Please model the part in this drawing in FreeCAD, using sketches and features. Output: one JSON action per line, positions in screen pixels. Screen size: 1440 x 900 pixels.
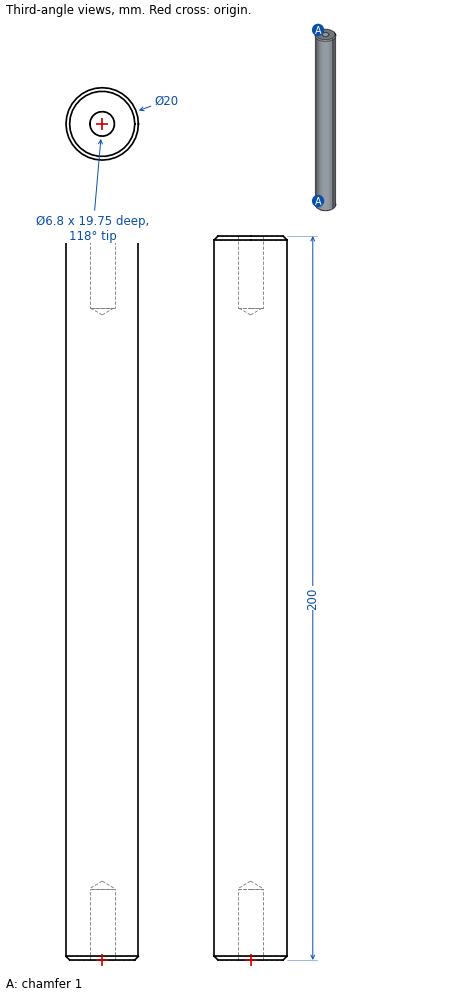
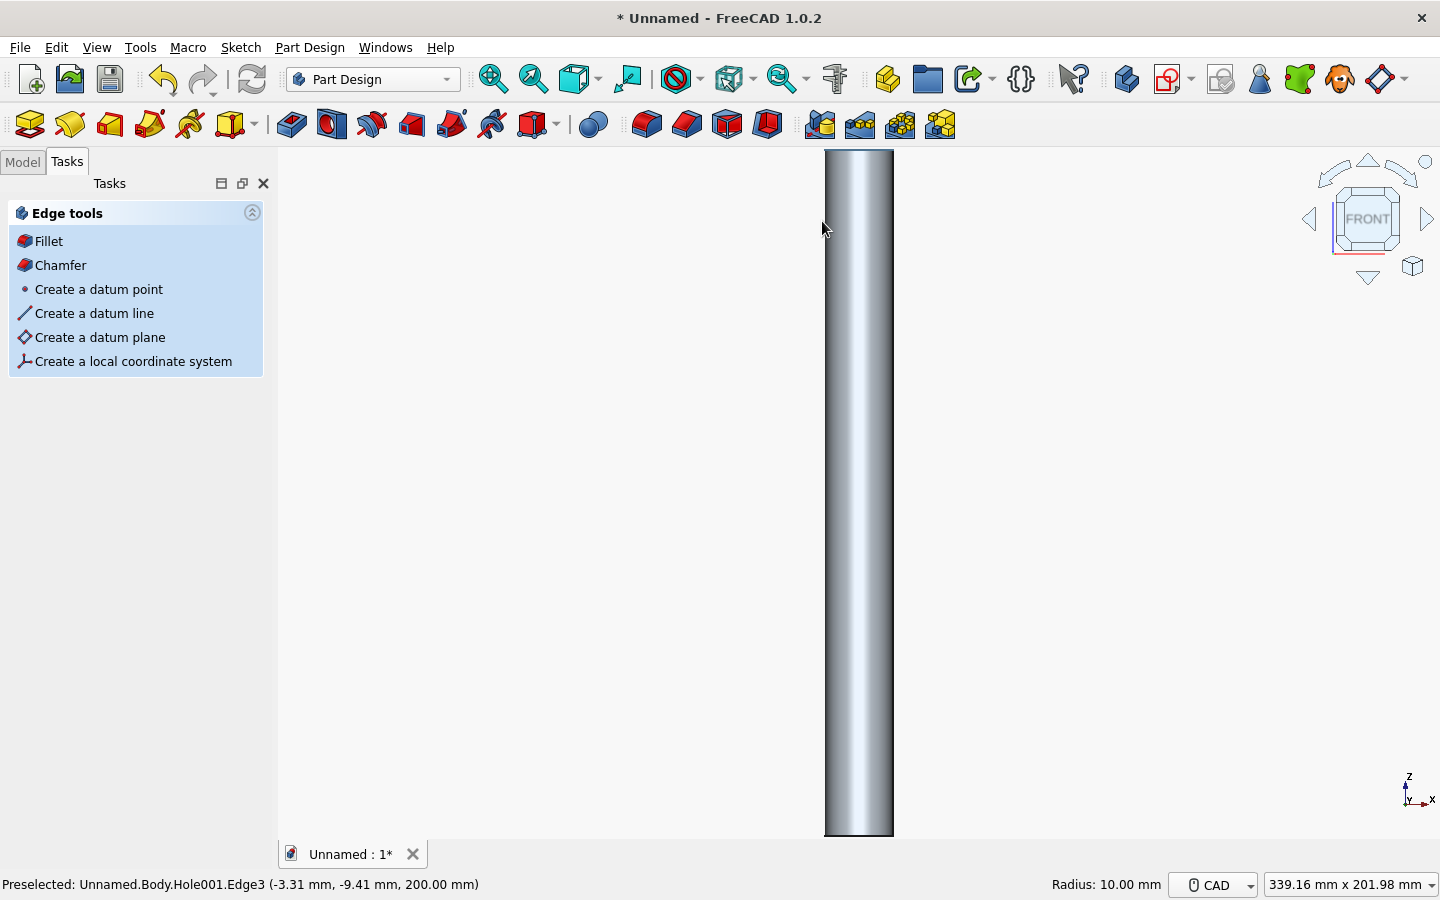
{"action": "key", "text": "3"}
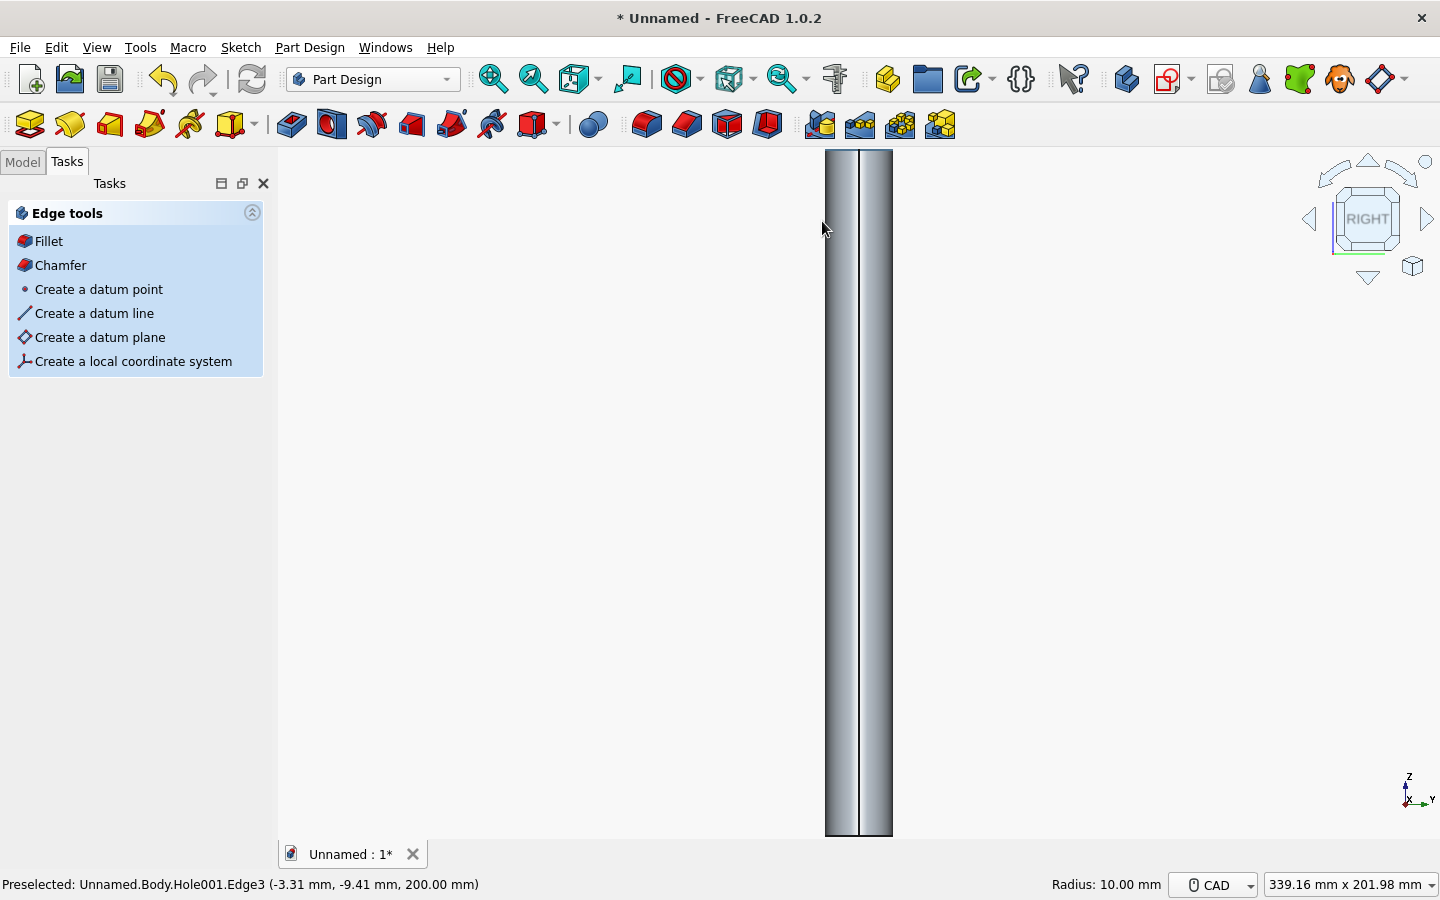
{"action": "key", "text": "5"}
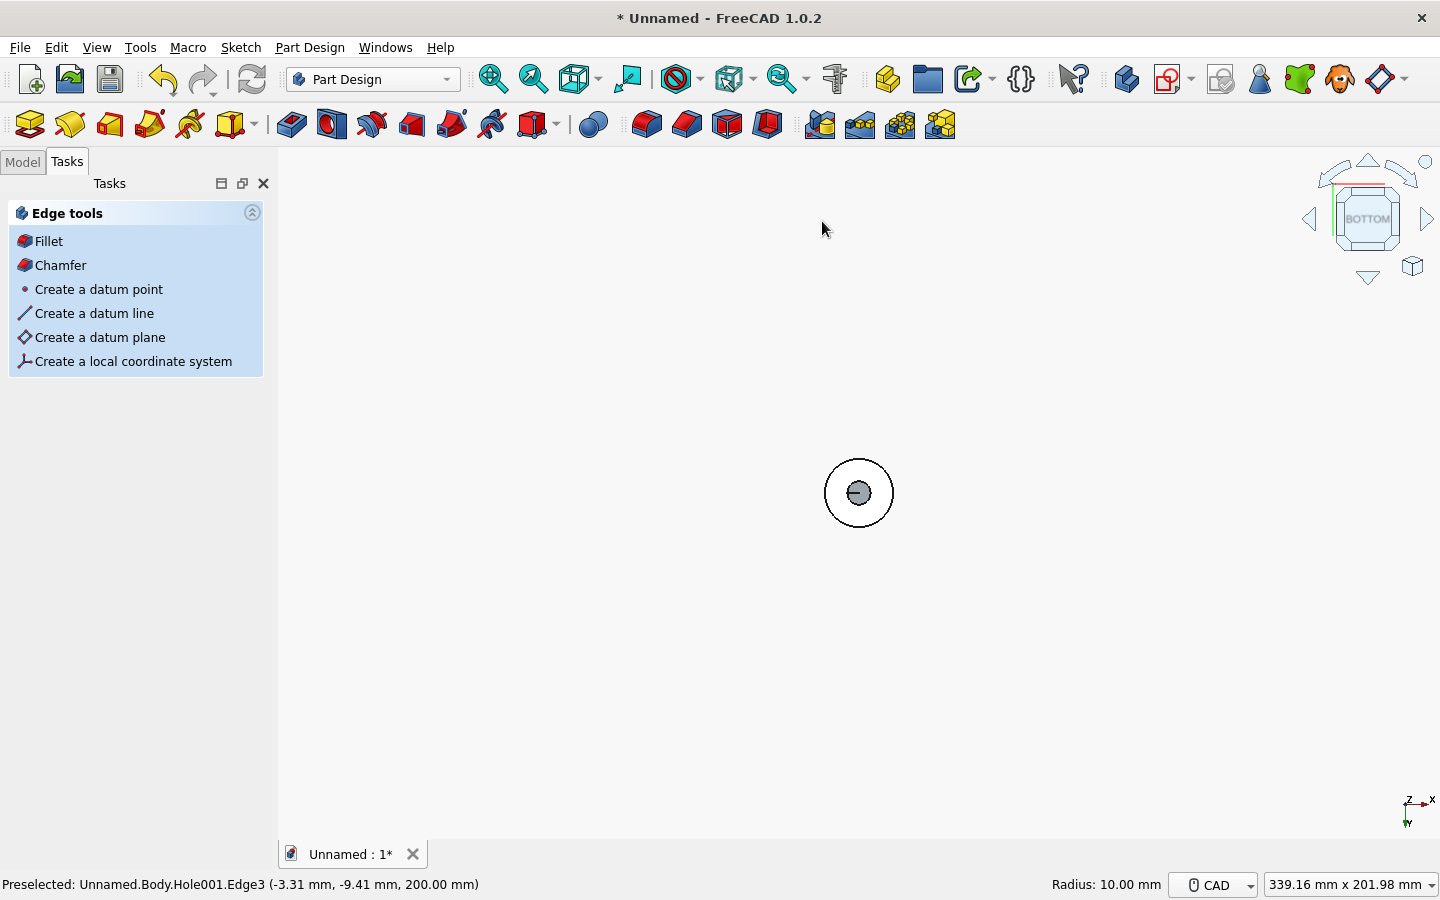
{"action": "left_click", "coordinate": [494, 80]}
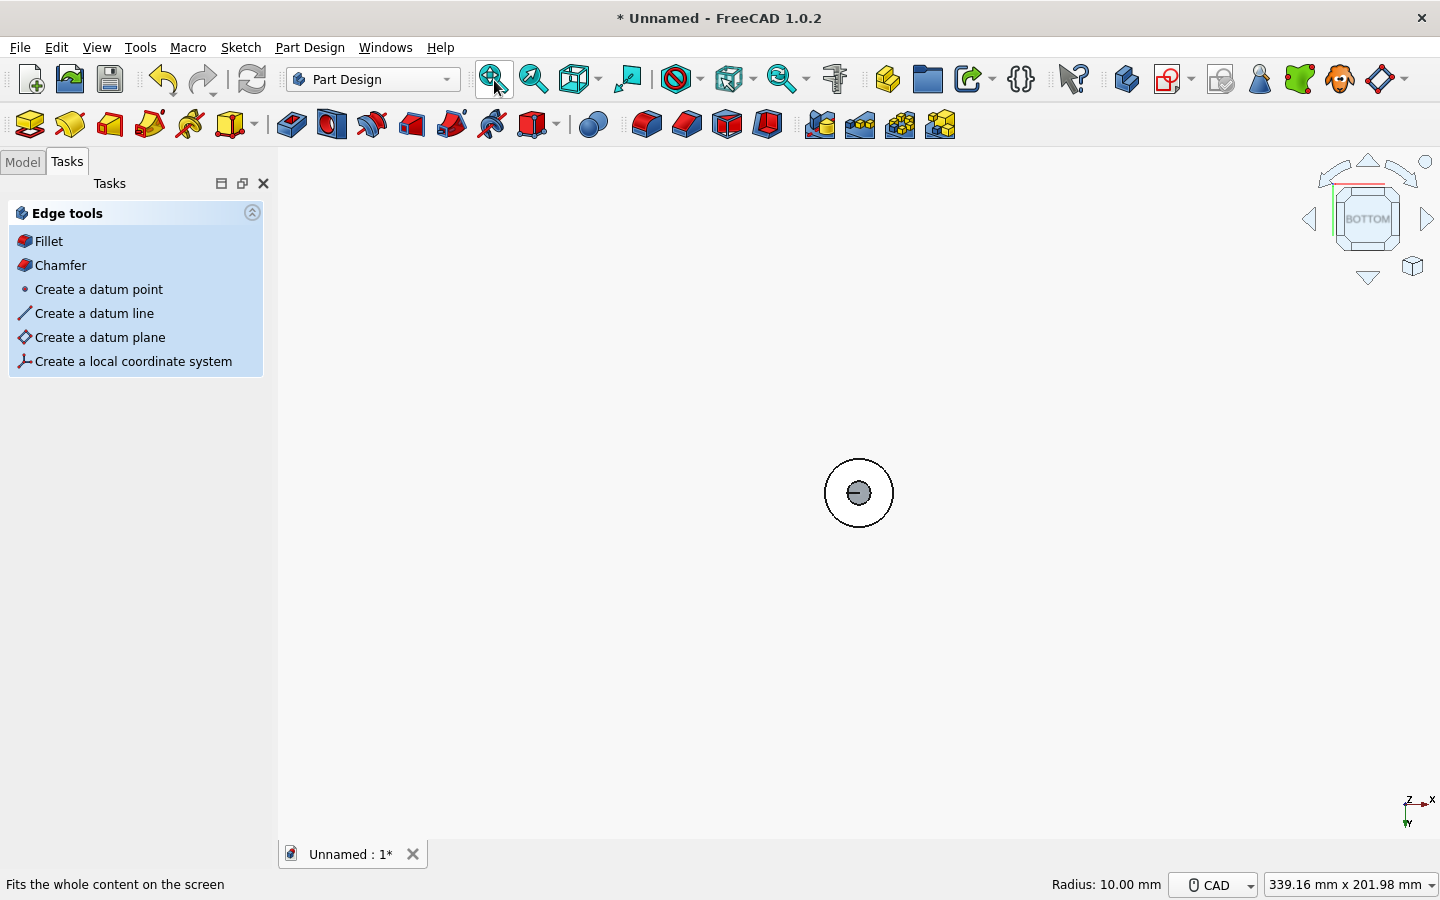
{"action": "left_click", "coordinate": [825, 492], "text": "ctrl"}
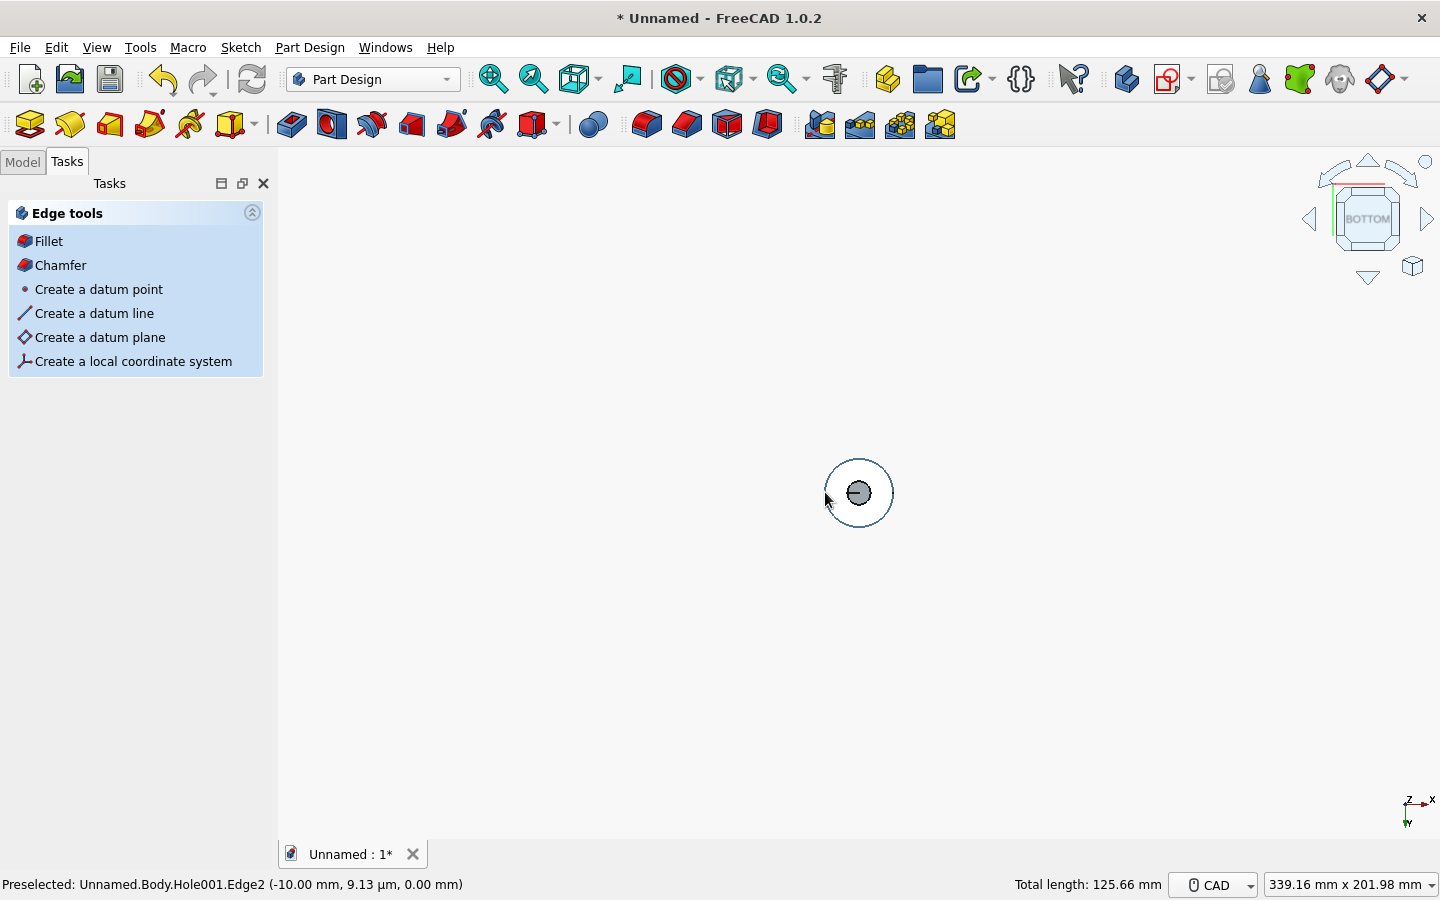
{"action": "left_click", "coordinate": [688, 124]}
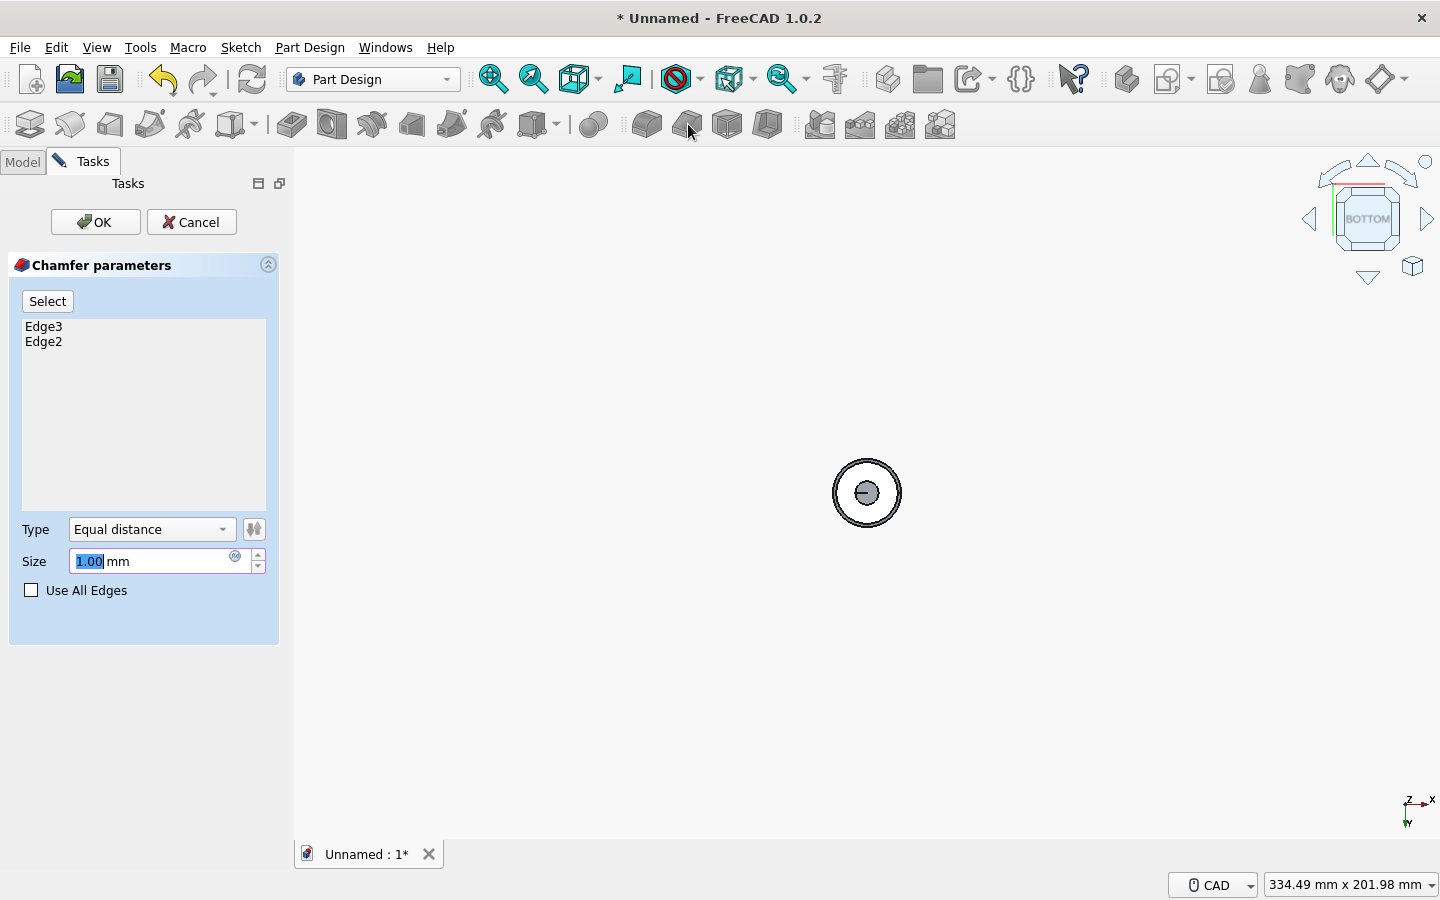
{"action": "type", "text": "1"}
{"action": "key", "text": "Tab"}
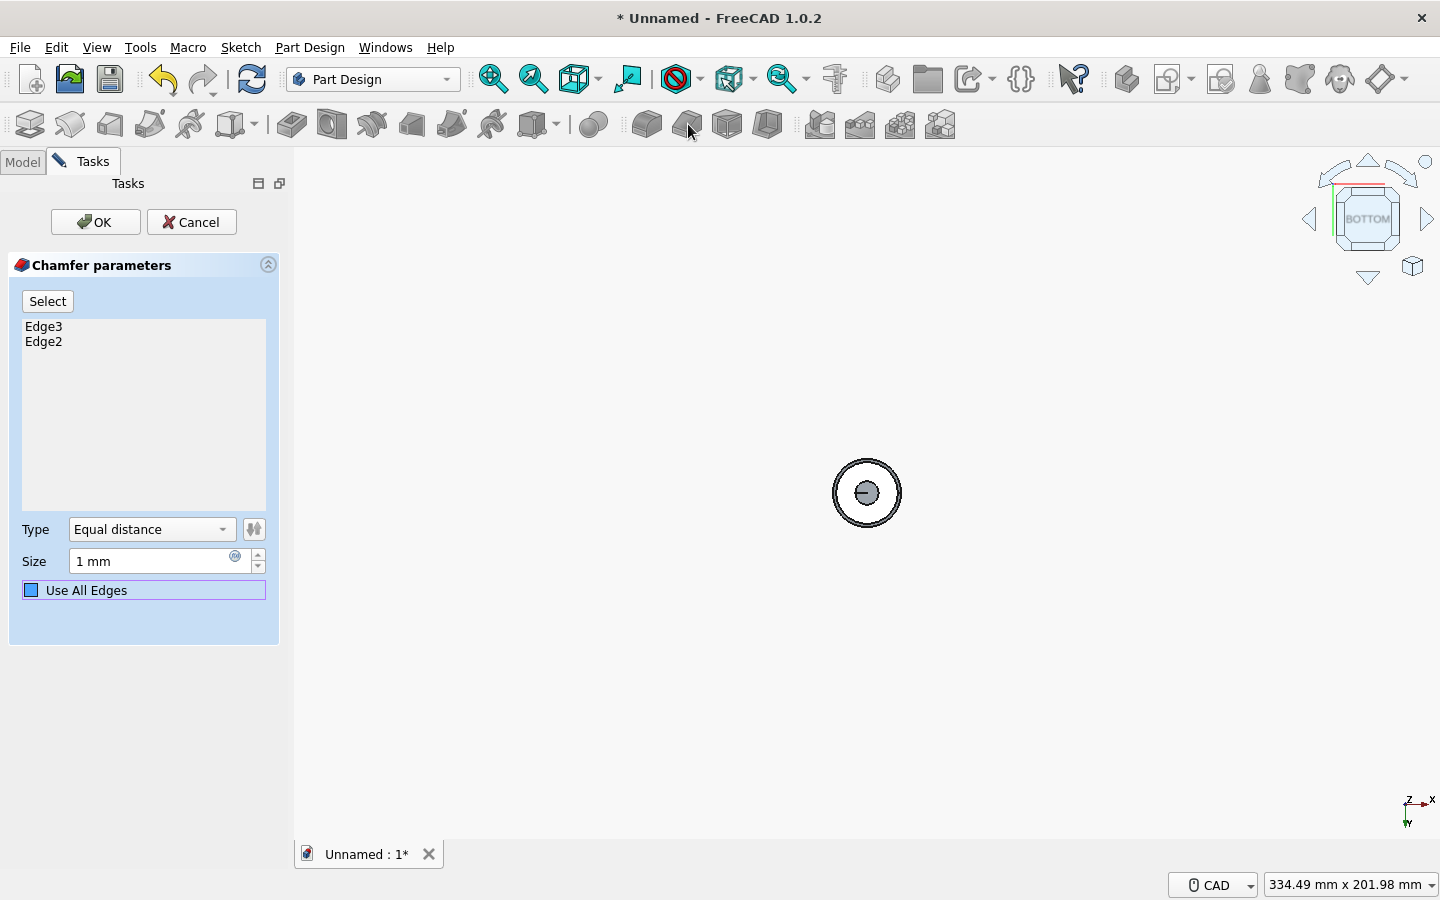
{"action": "left_click", "coordinate": [96, 222]}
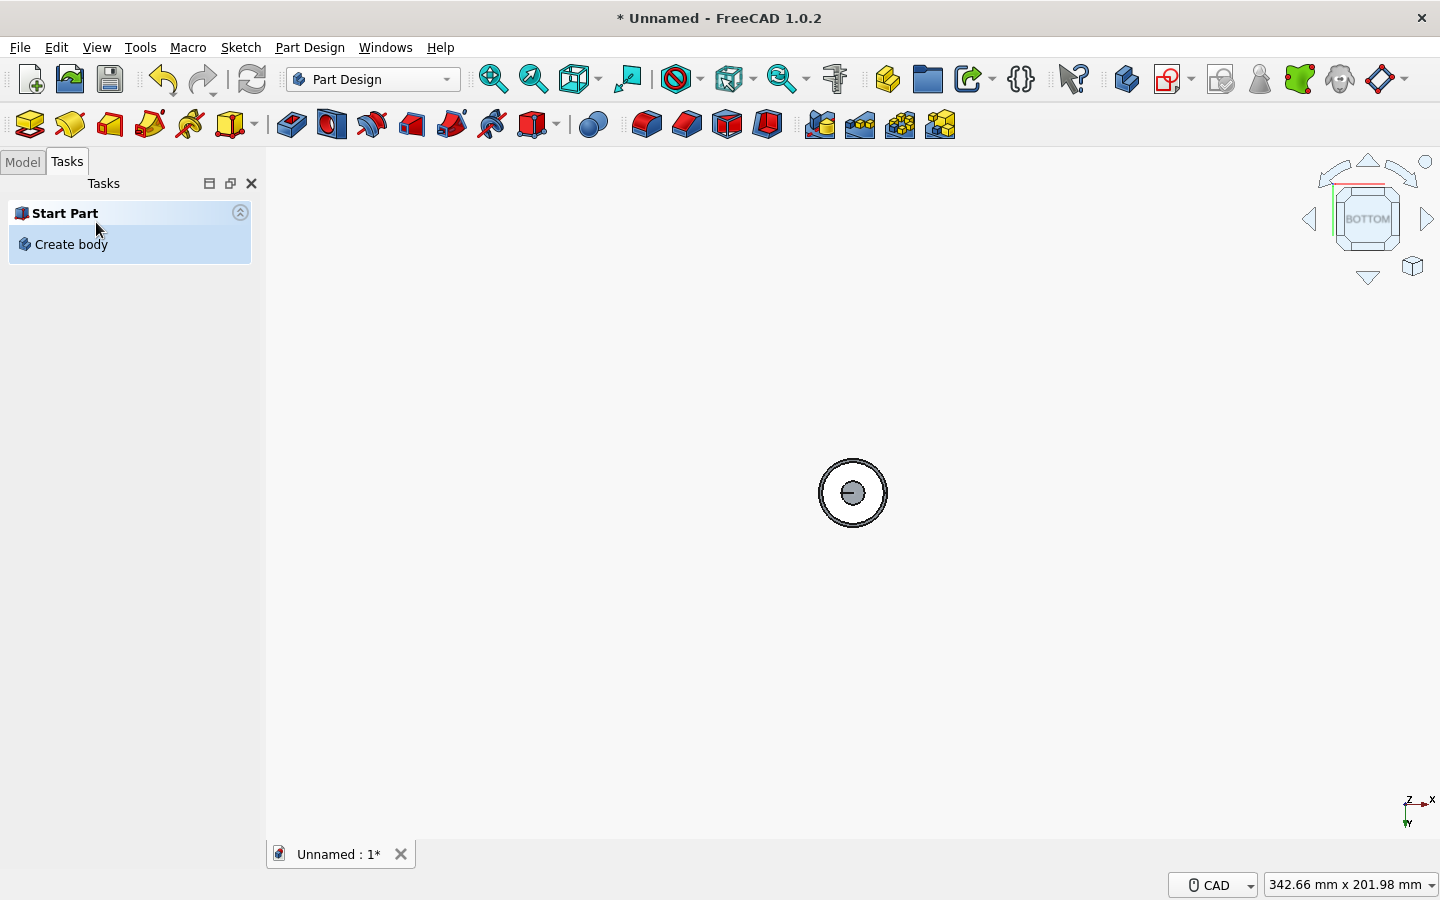
{"action": "key", "text": "0"}